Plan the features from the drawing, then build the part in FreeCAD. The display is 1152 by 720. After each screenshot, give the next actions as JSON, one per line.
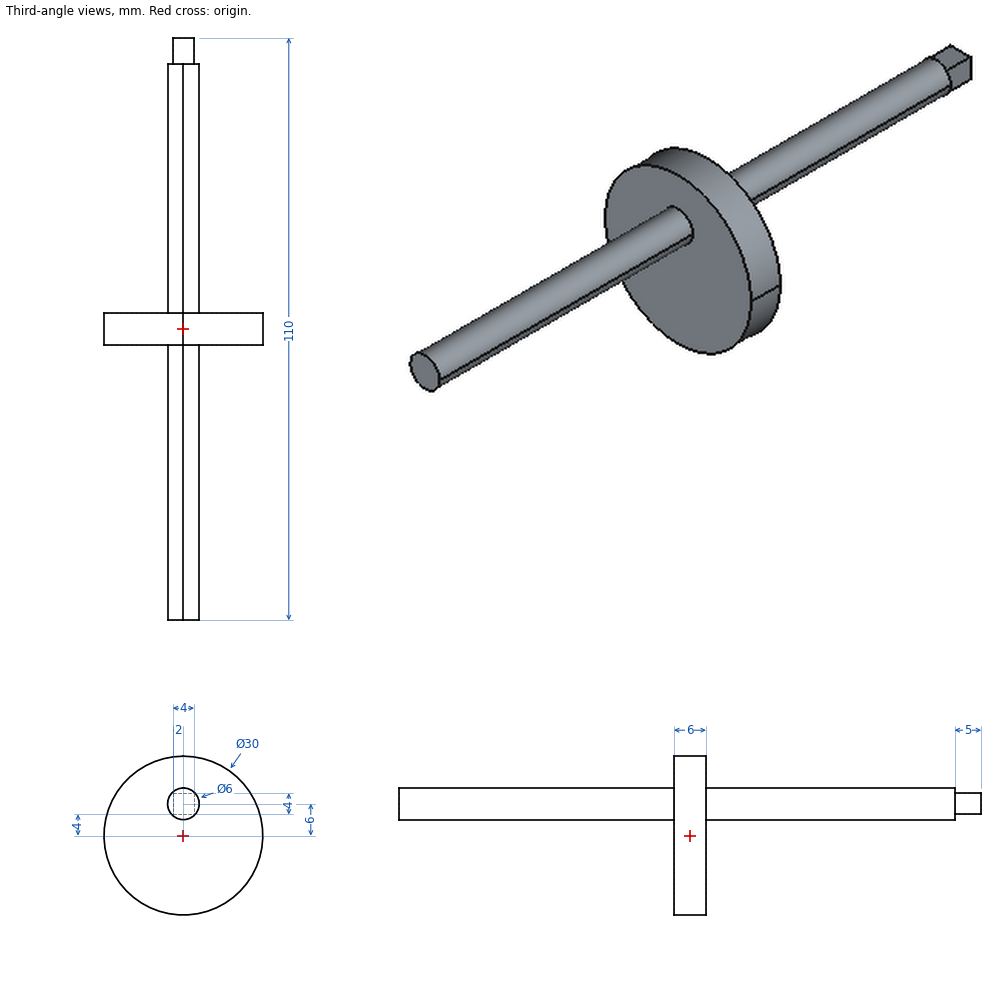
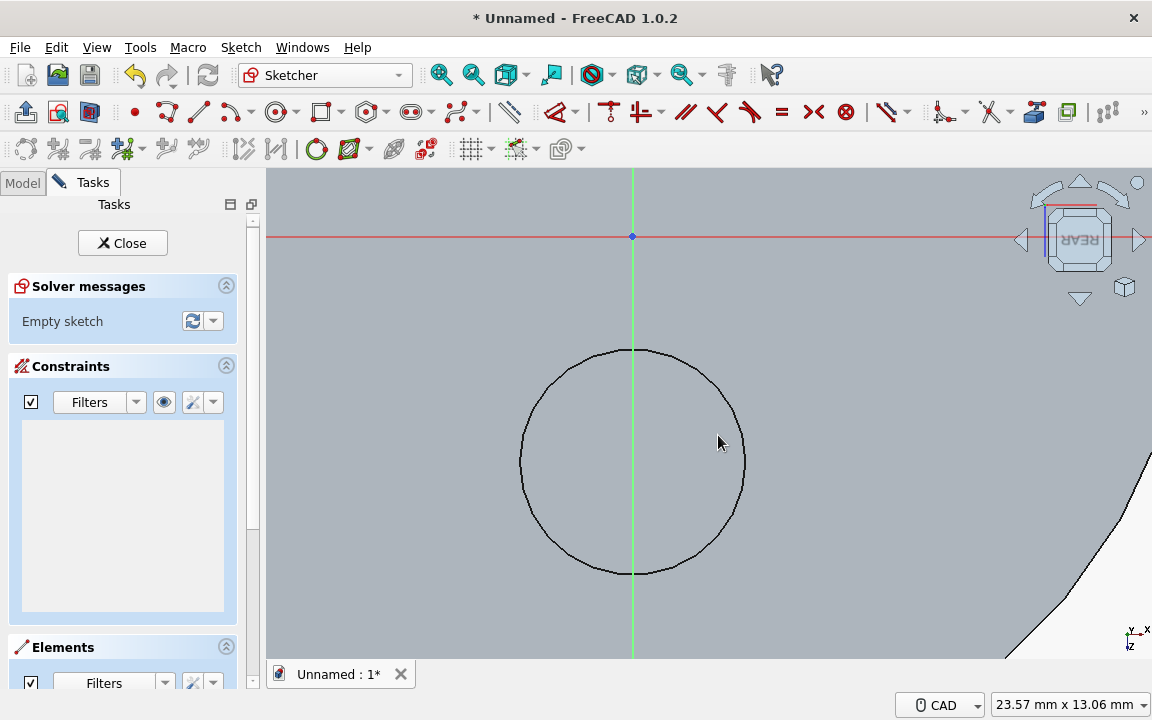
{"action": "key", "text": "g r"}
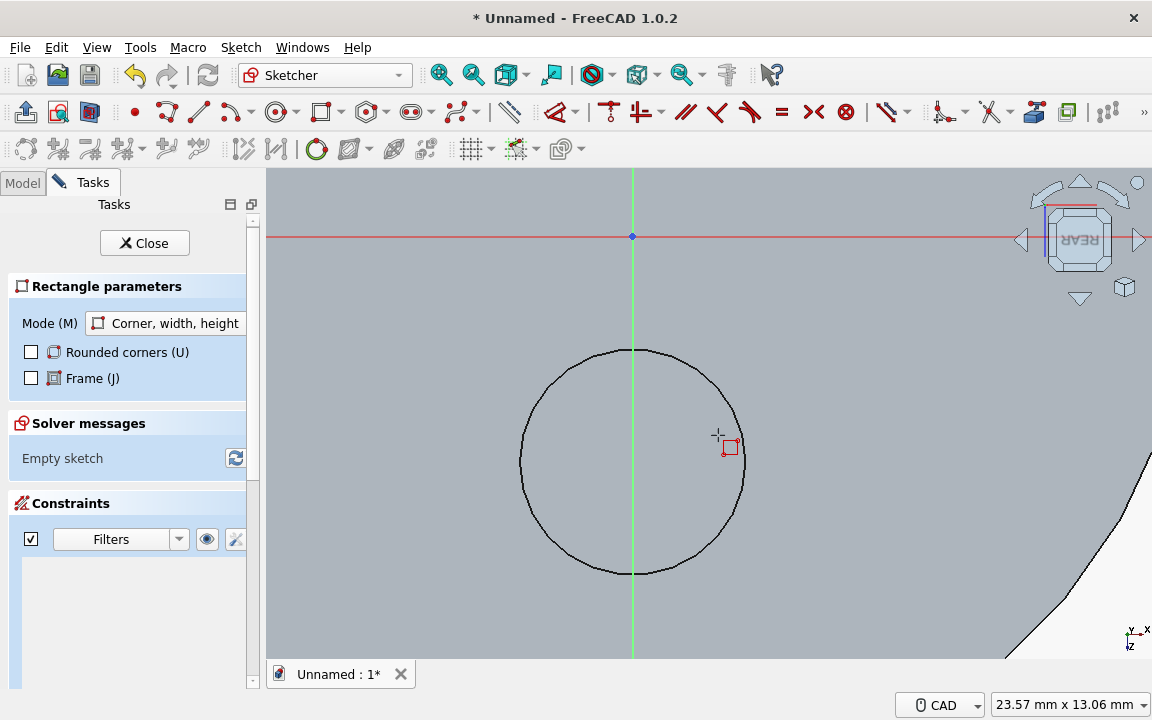
{"action": "left_click", "coordinate": [558, 387]}
{"action": "mouse_move", "coordinate": [708, 537]}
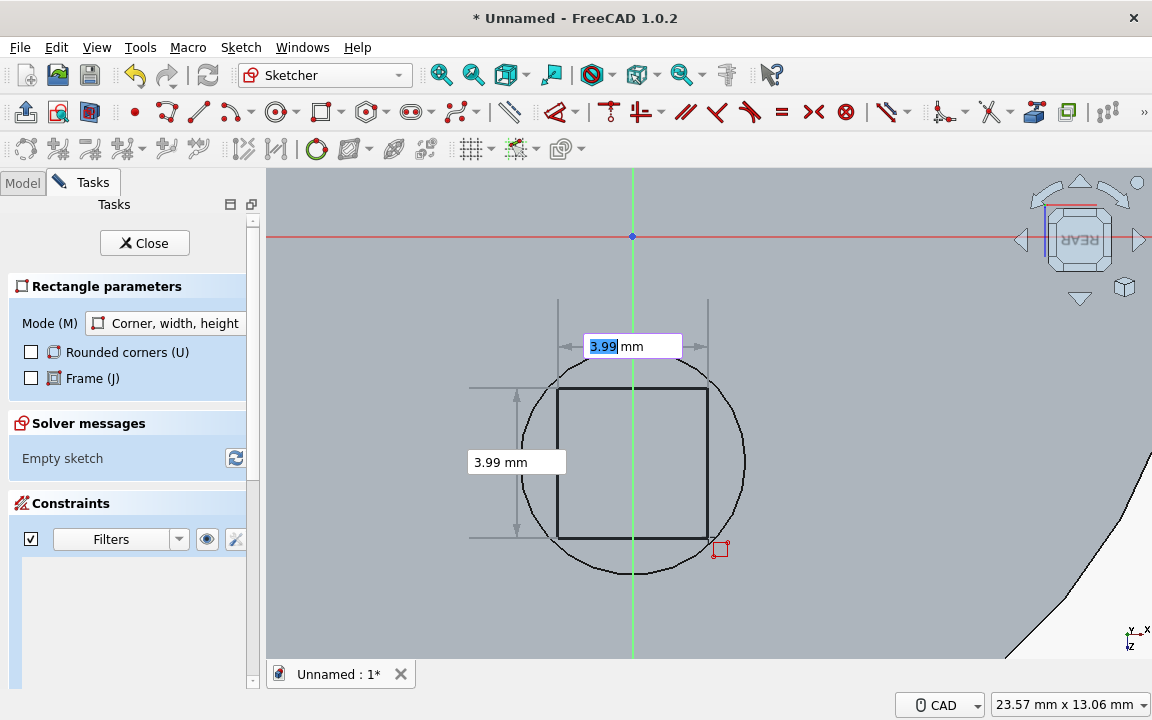
{"action": "type", "text": "4"}
{"action": "key", "text": "Tab"}
{"action": "type", "text": "4"}
{"action": "key", "text": "Return"}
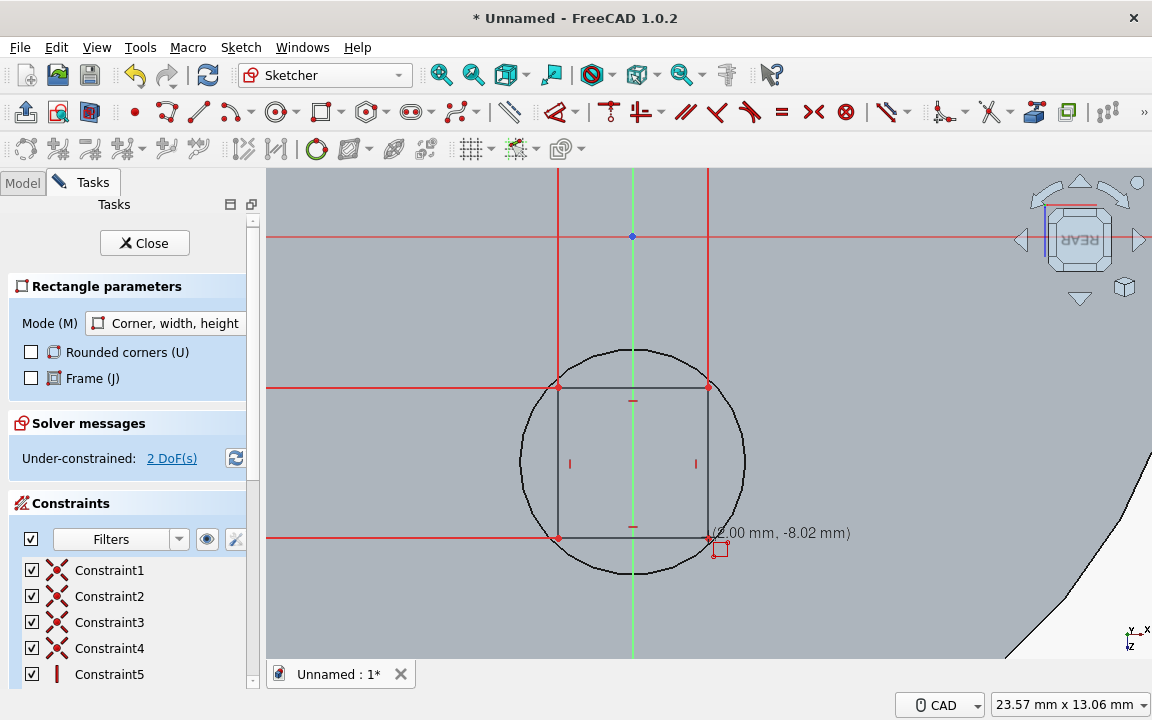
{"action": "left_click", "coordinate": [276, 112]}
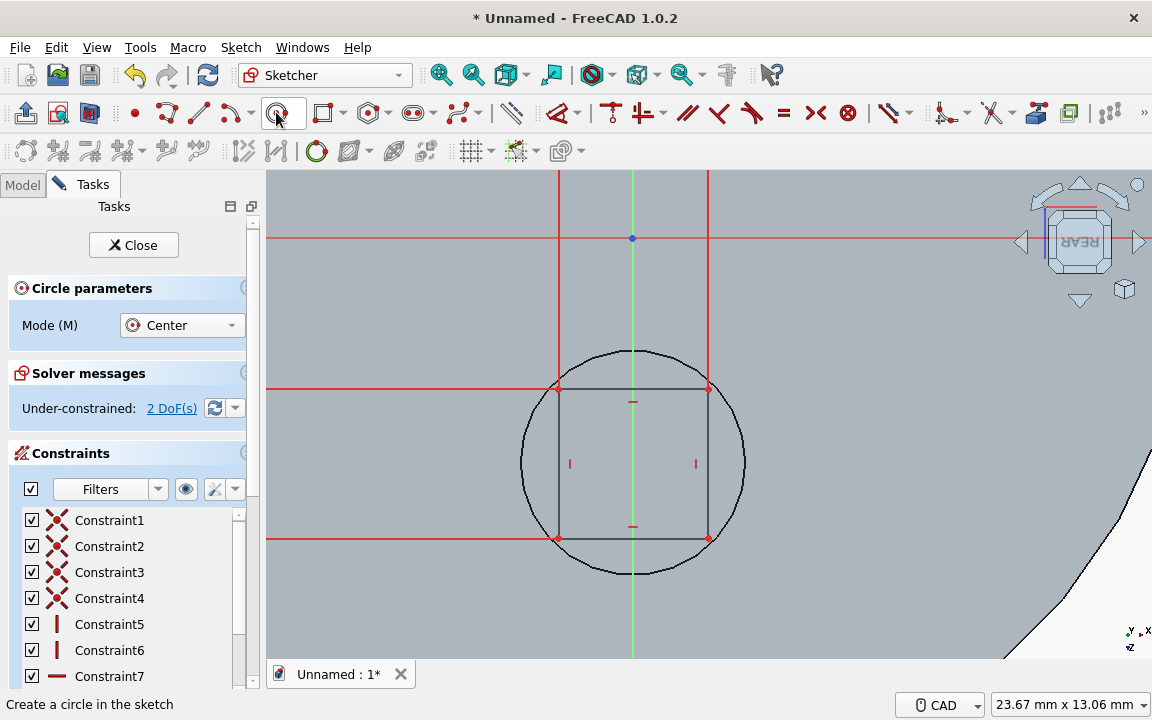
{"action": "left_click", "coordinate": [633, 463]}
{"action": "mouse_move", "coordinate": [739, 424]}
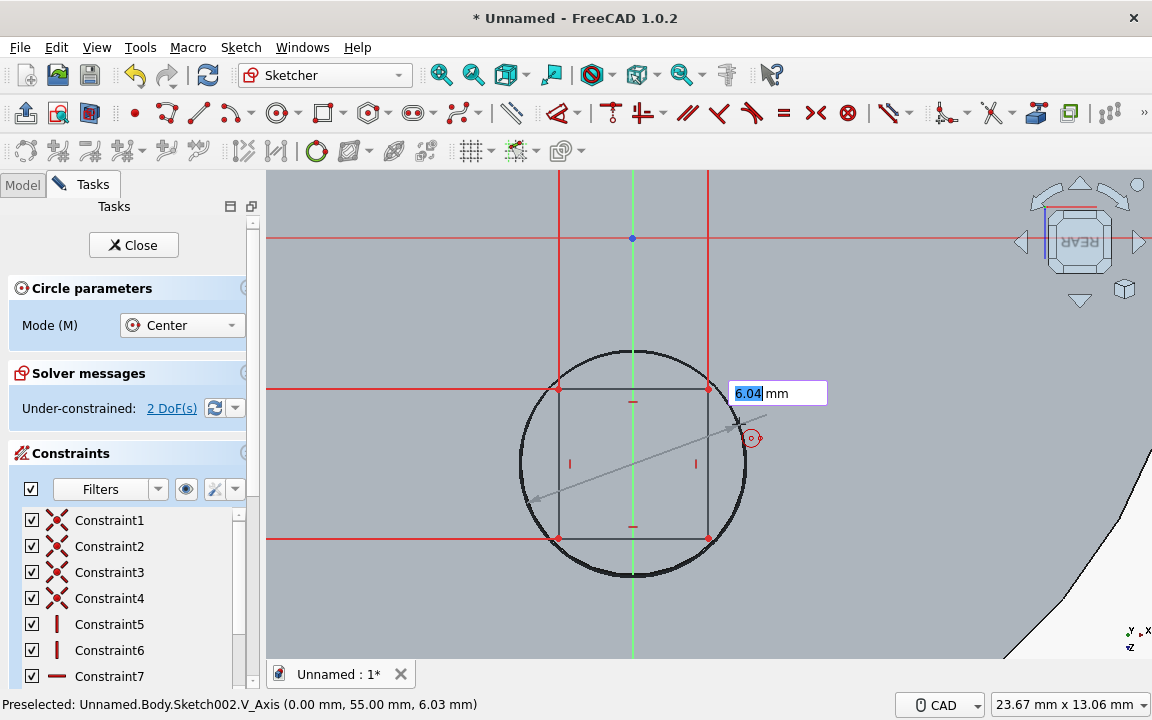
{"action": "type", "text": "6"}
{"action": "key", "text": "Return"}
{"action": "key", "text": "Escape"}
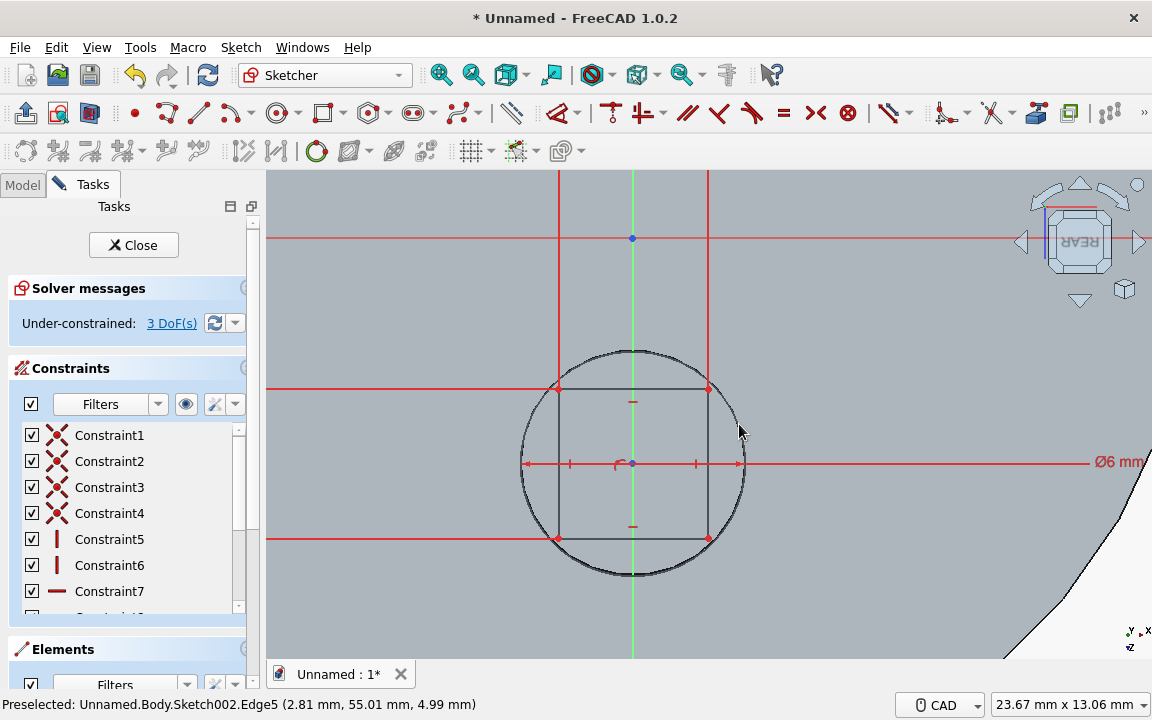
{"action": "left_click", "coordinate": [633, 464]}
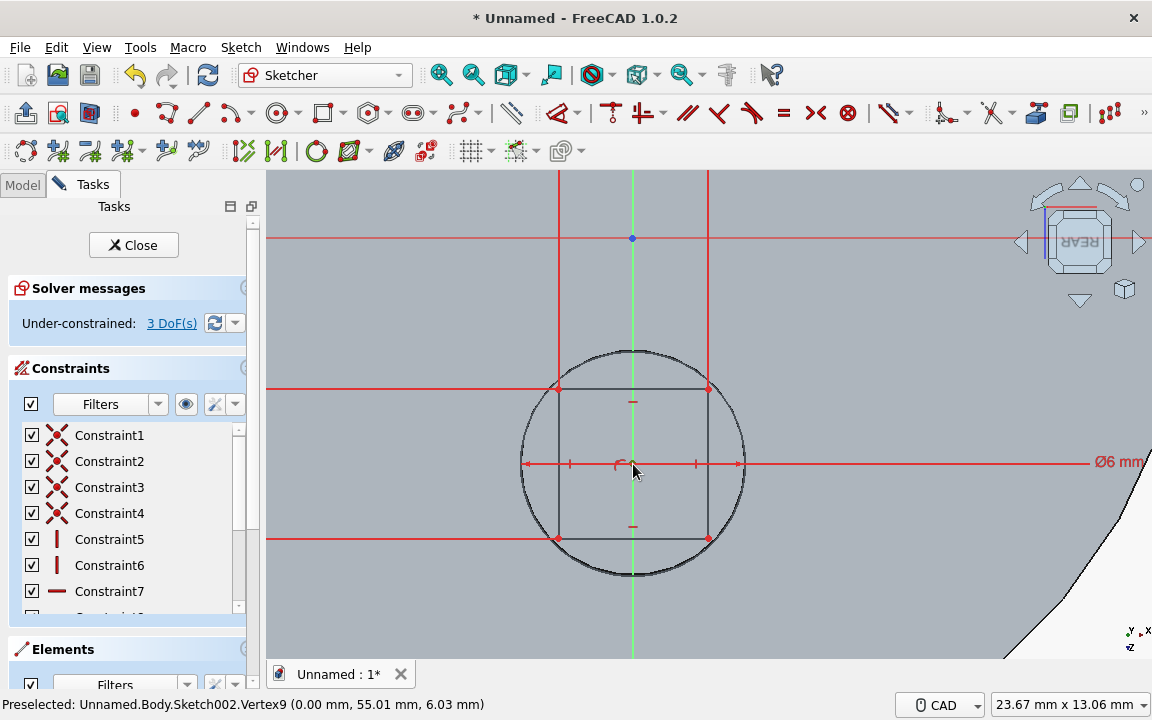
{"action": "key", "text": "i"}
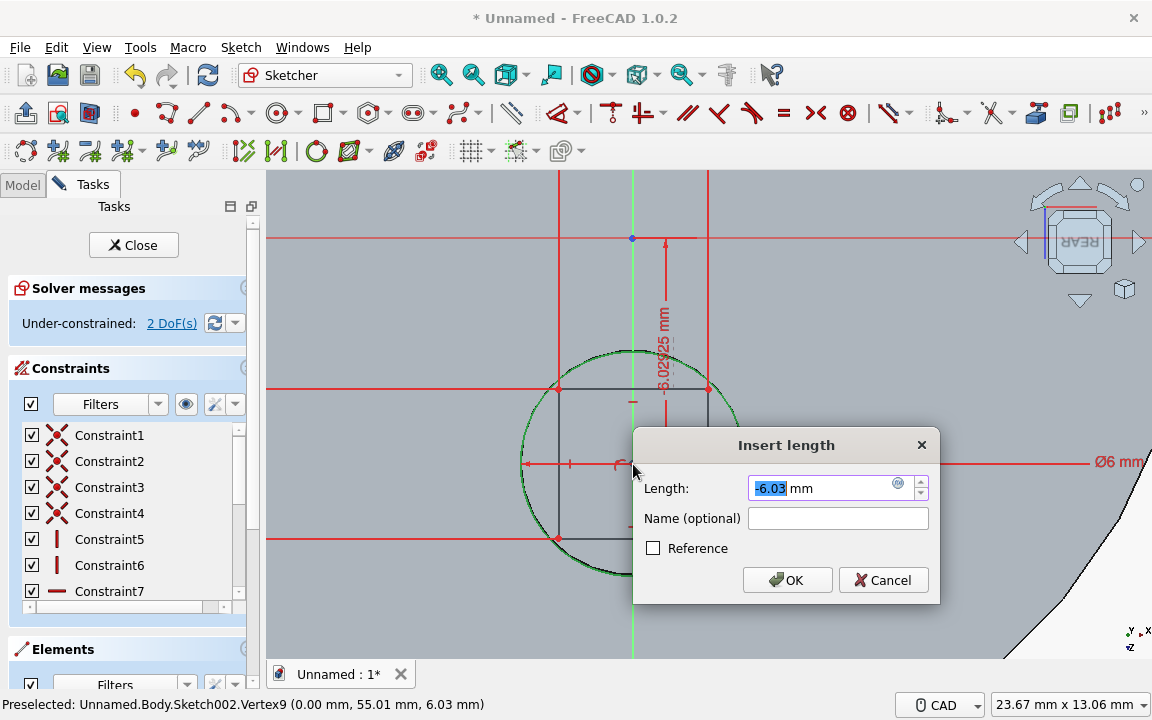
{"action": "type", "text": "-6"}
{"action": "key", "text": "Return"}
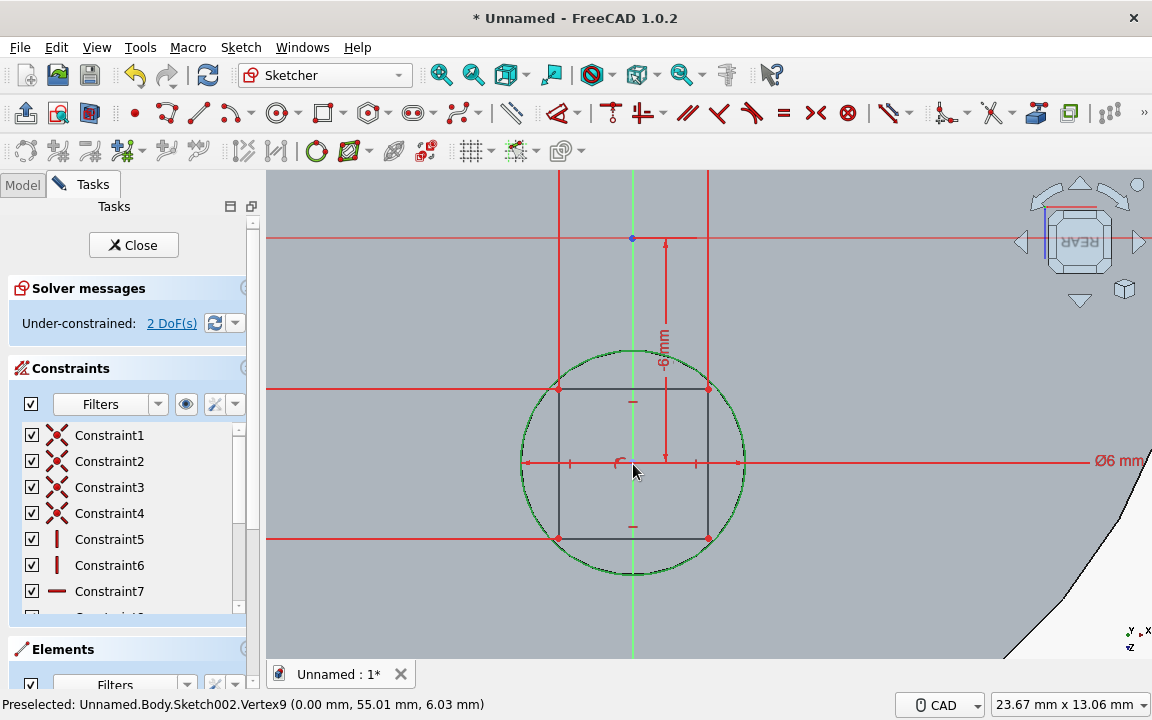
{"action": "left_click", "coordinate": [559, 389]}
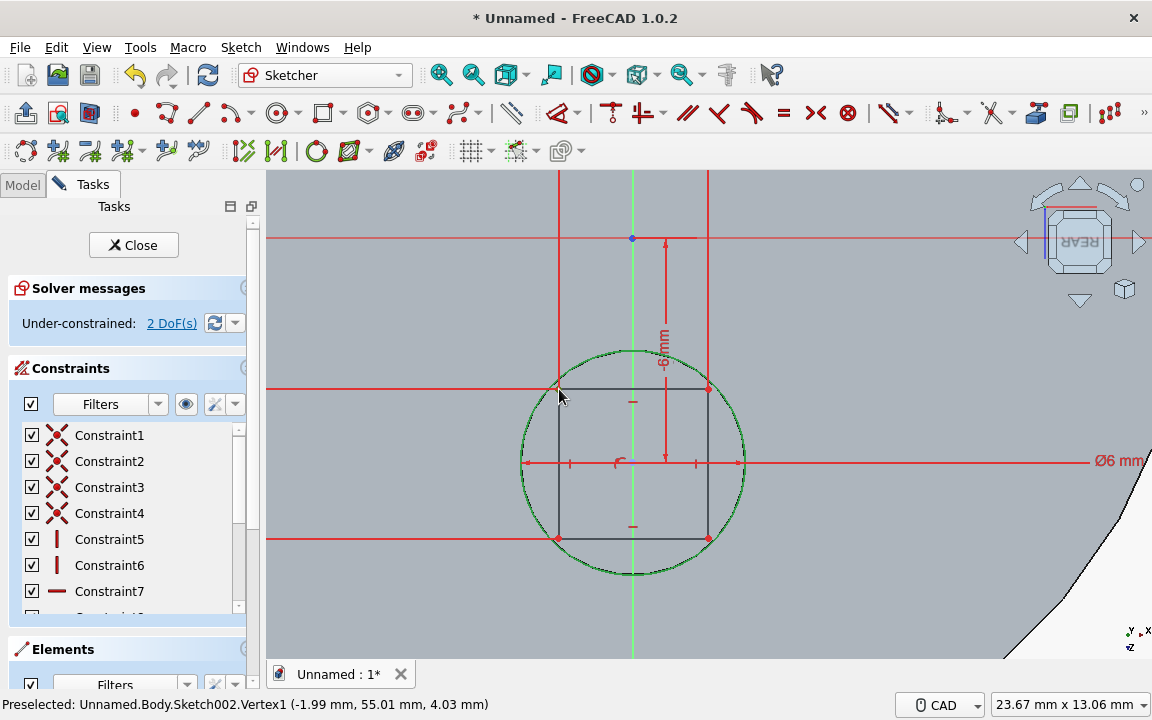
{"action": "key", "text": "l"}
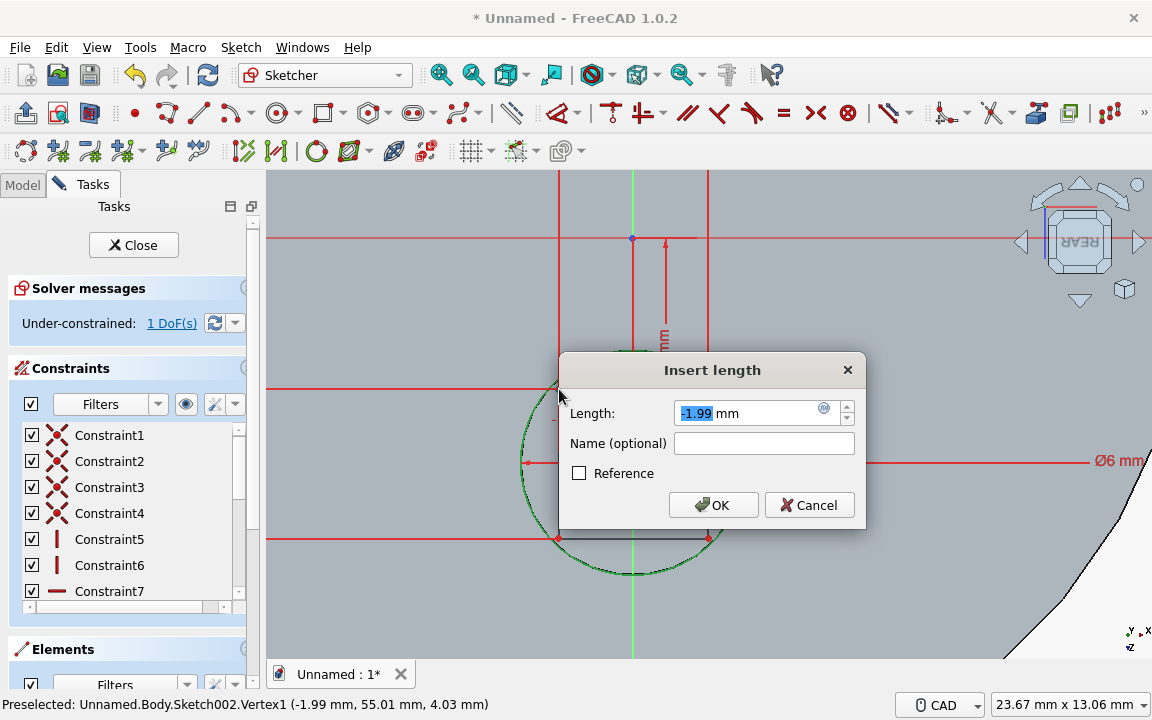
{"action": "type", "text": "-2"}
{"action": "key", "text": "Return"}